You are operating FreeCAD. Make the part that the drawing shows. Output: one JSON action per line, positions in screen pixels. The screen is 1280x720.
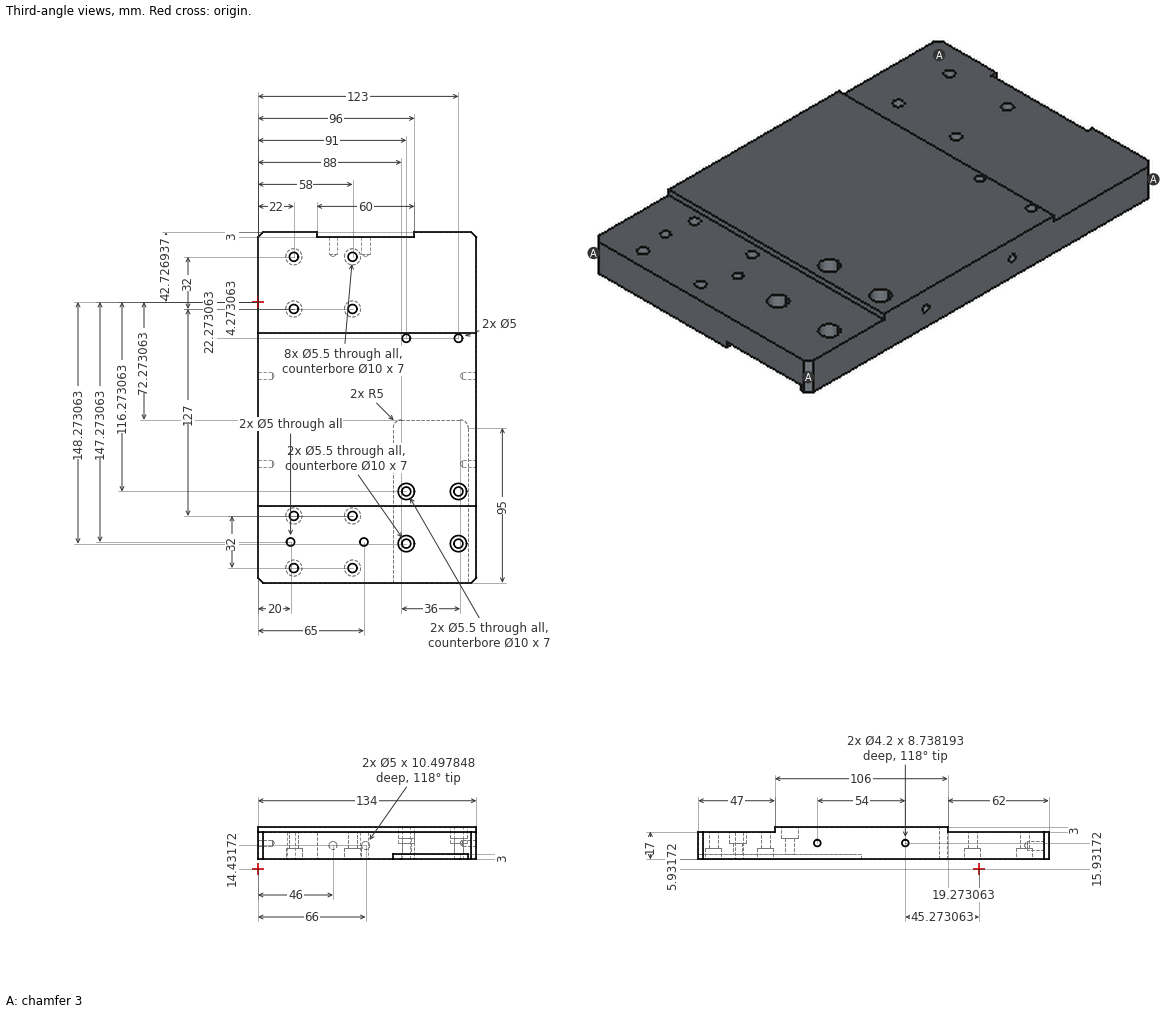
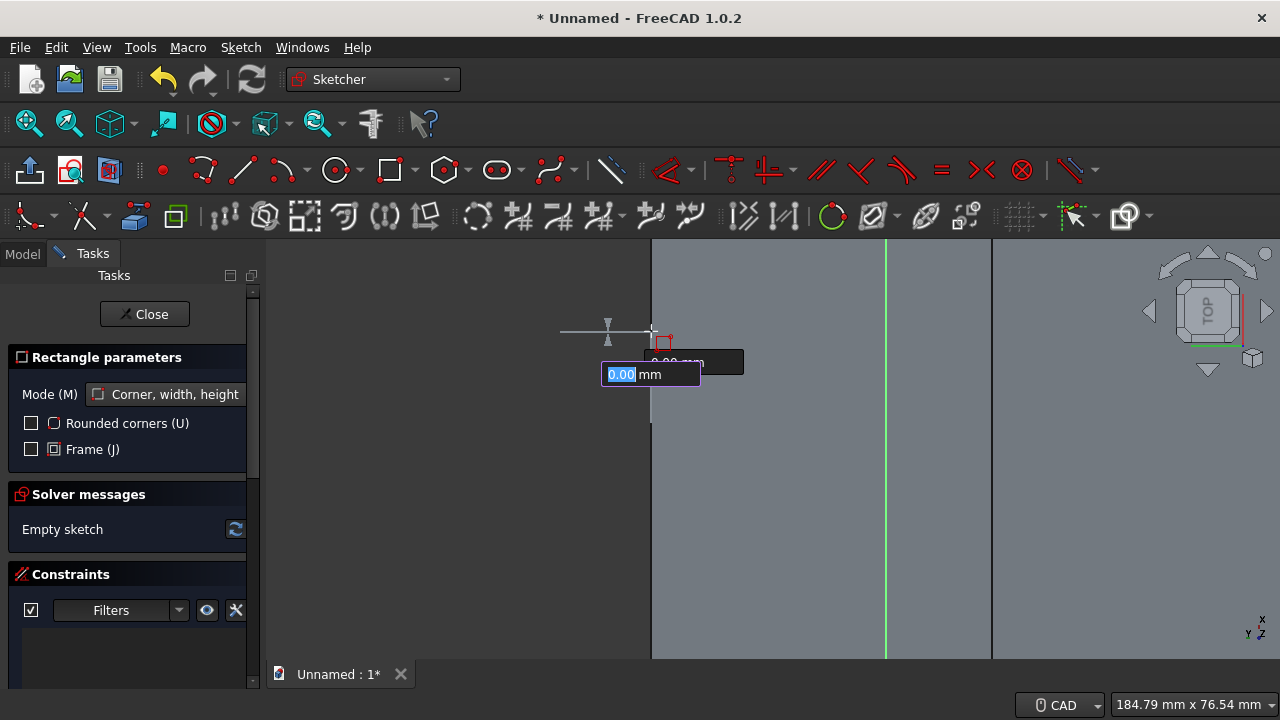
{"action": "scroll", "coordinate": [652, 331], "scroll_direction": "down", "scroll_amount": 4}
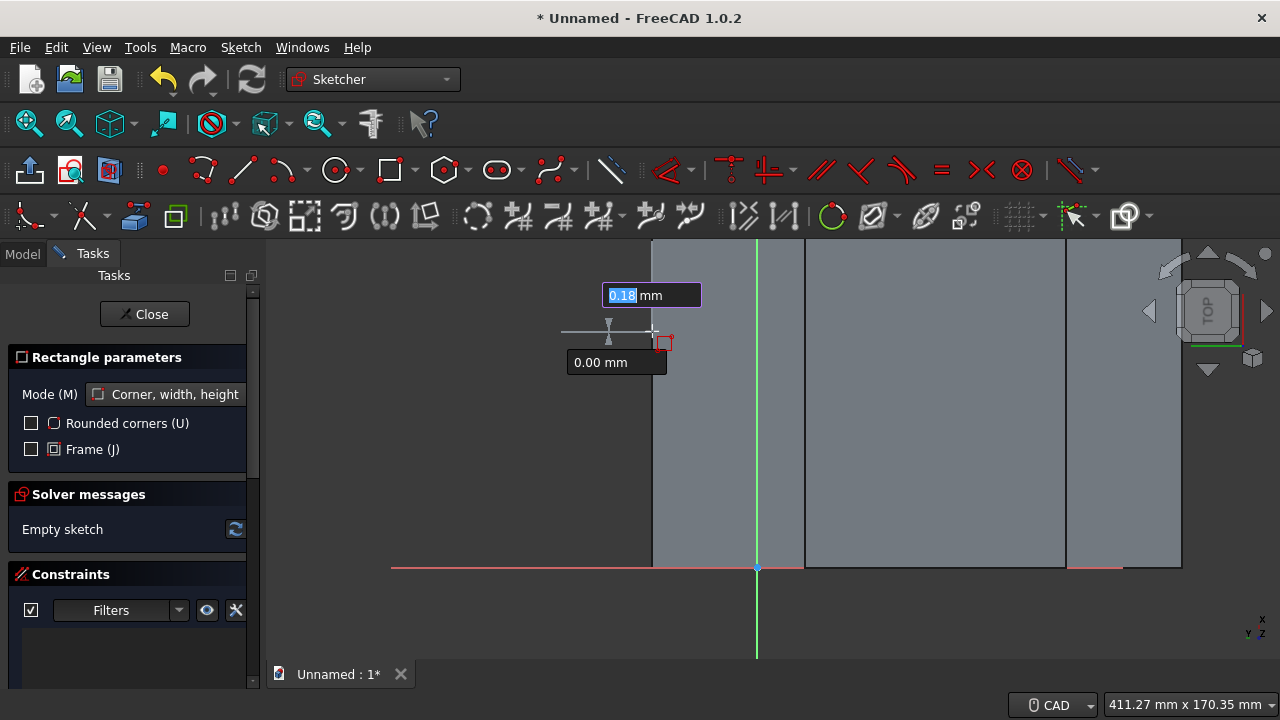
{"action": "left_click", "coordinate": [659, 479]}
{"action": "key", "text": "Escape"}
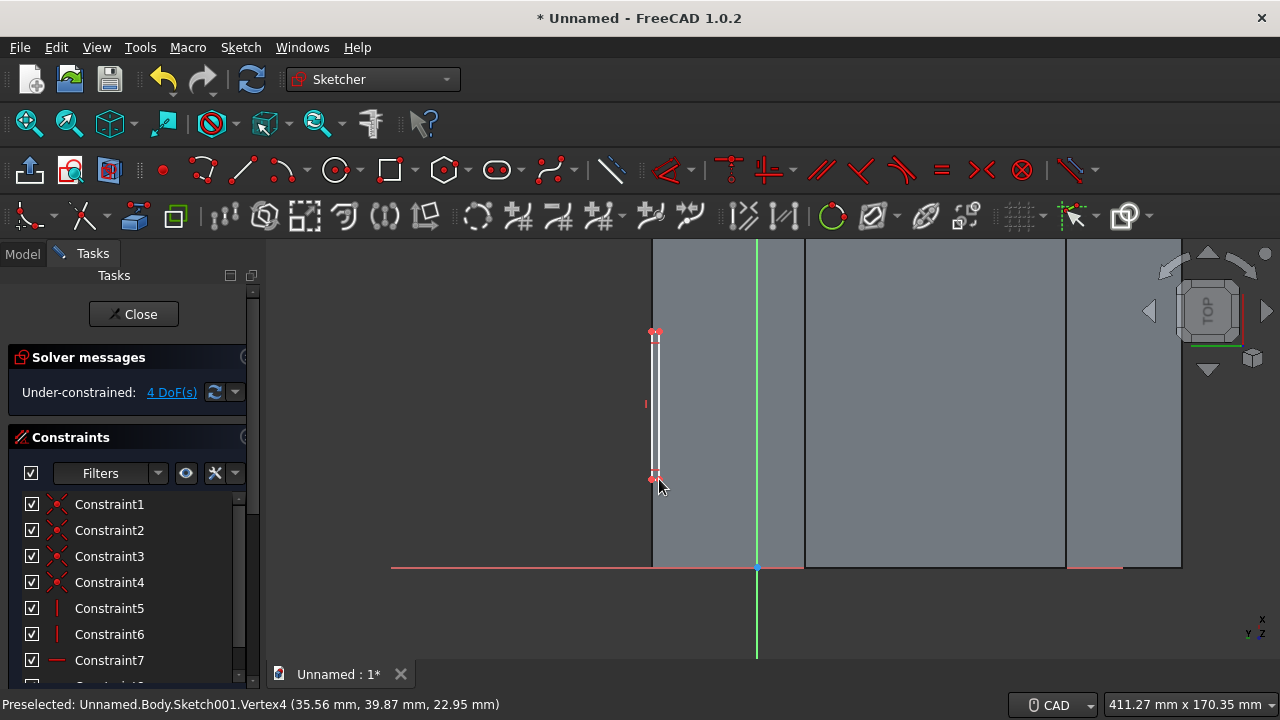
{"action": "left_click", "coordinate": [666, 170]}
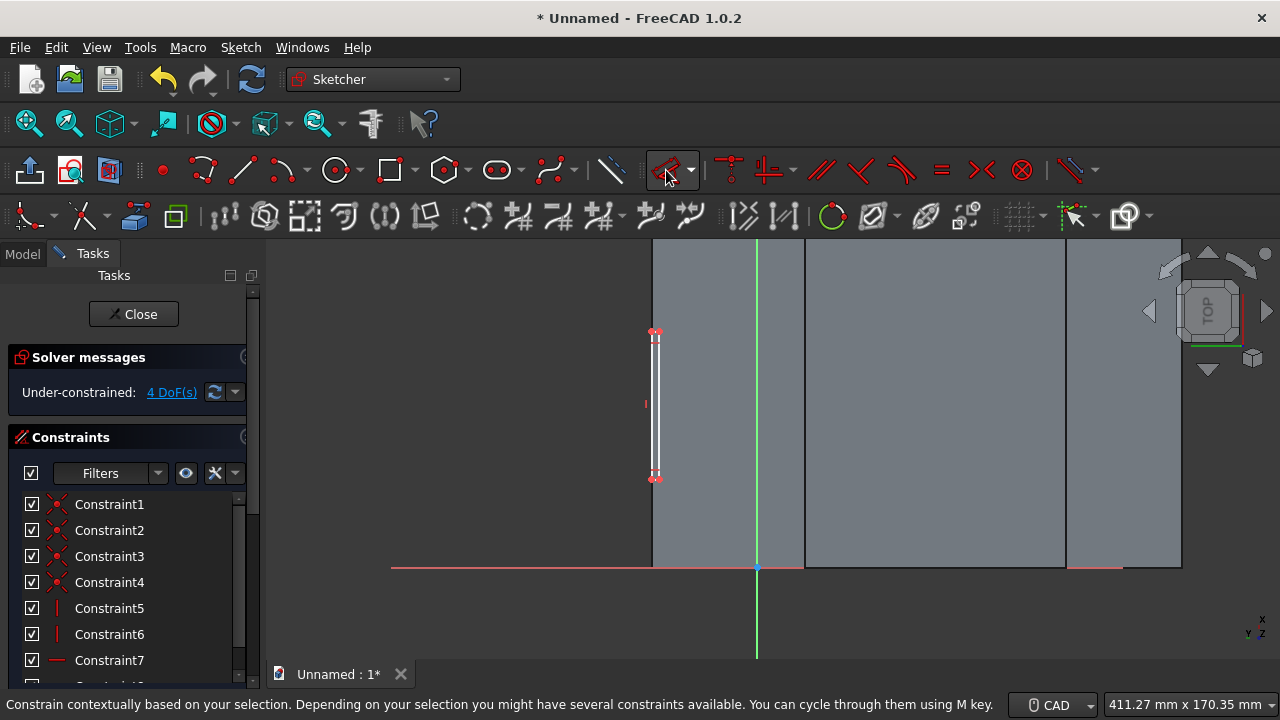
{"action": "scroll", "coordinate": [655, 480], "scroll_direction": "up", "scroll_amount": 9}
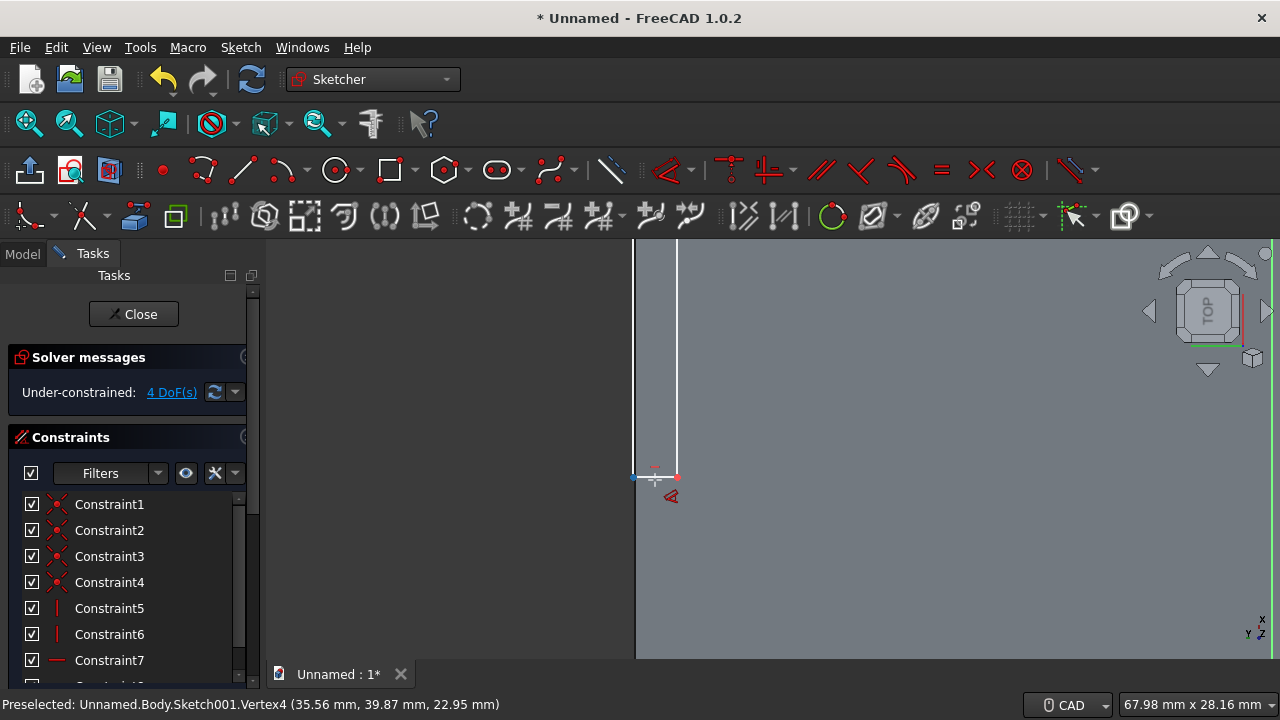
{"action": "left_click", "coordinate": [655, 477]}
{"action": "left_click", "coordinate": [655, 511]}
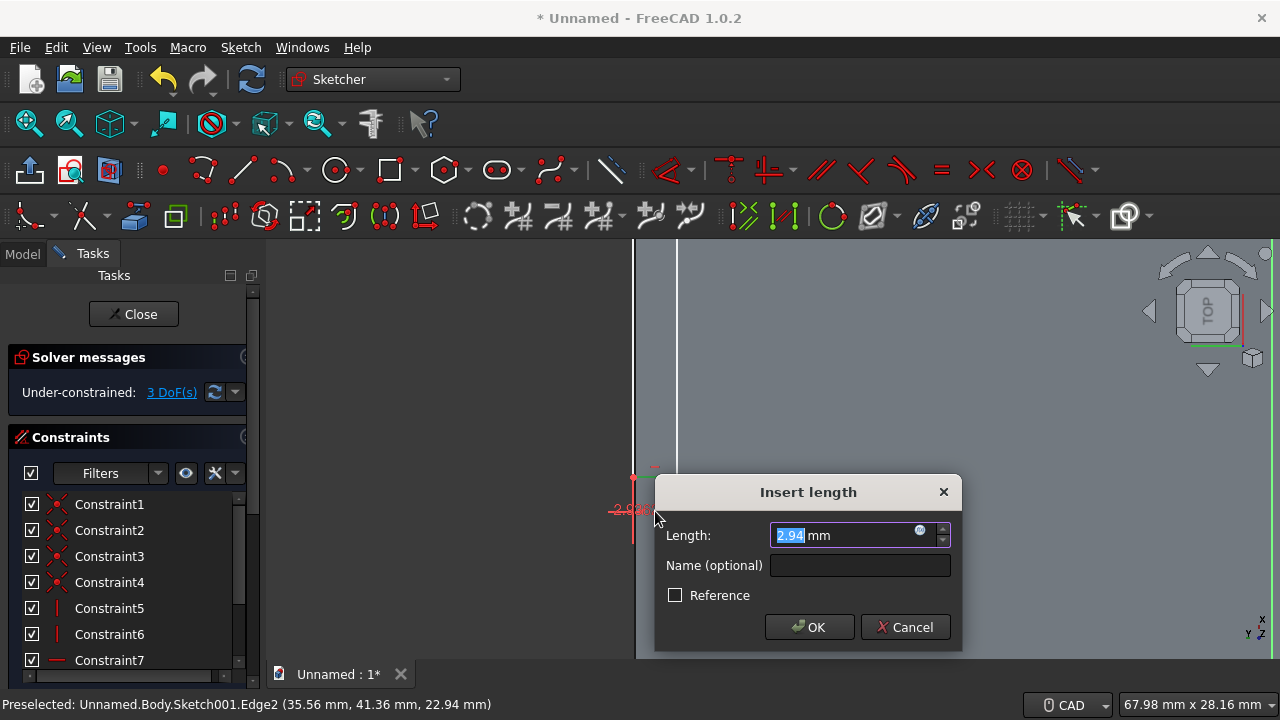
{"action": "type", "text": "3"}
{"action": "key", "text": "Return"}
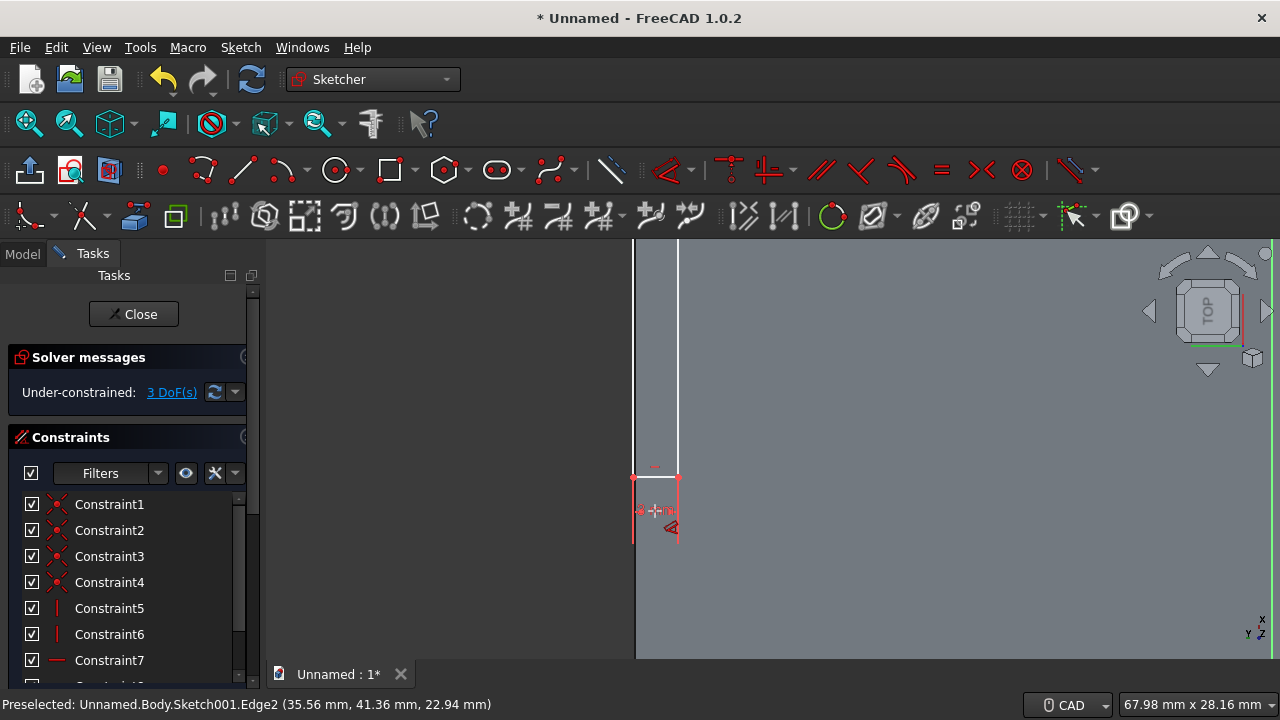
{"action": "scroll", "coordinate": [655, 480], "scroll_direction": "down", "scroll_amount": 9}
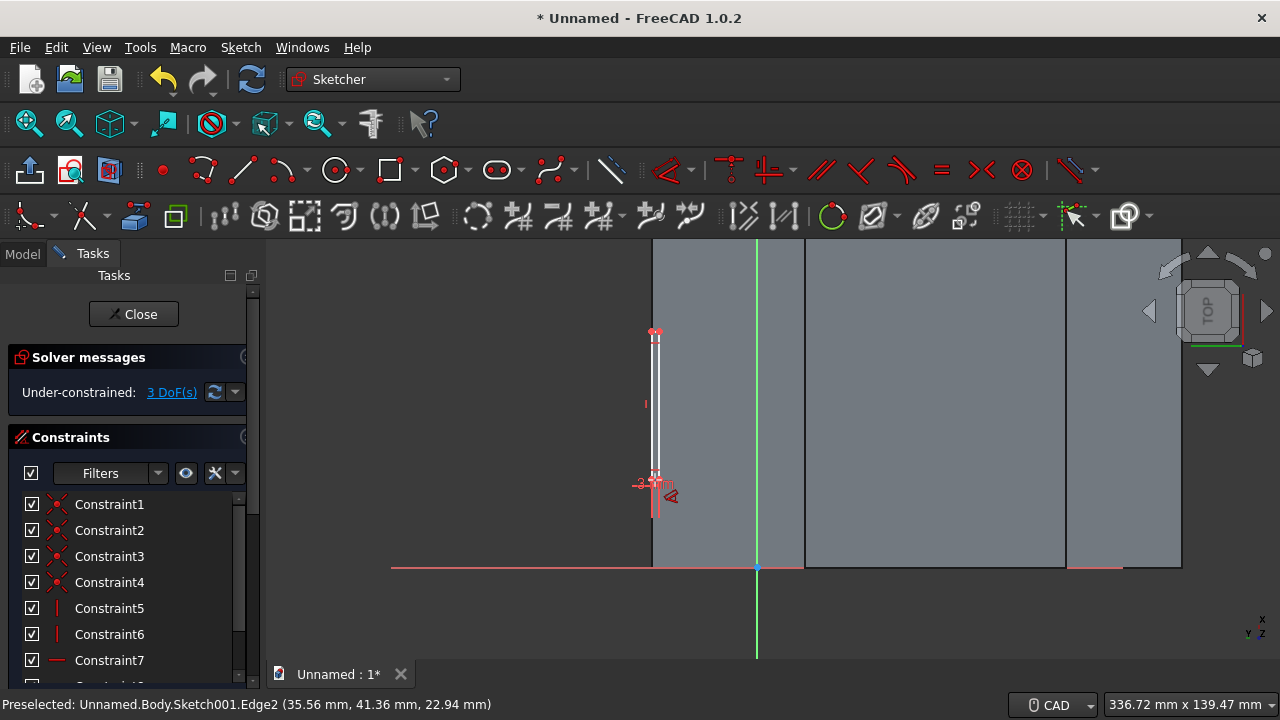
{"action": "scroll", "coordinate": [652, 450], "scroll_direction": "up", "scroll_amount": 4}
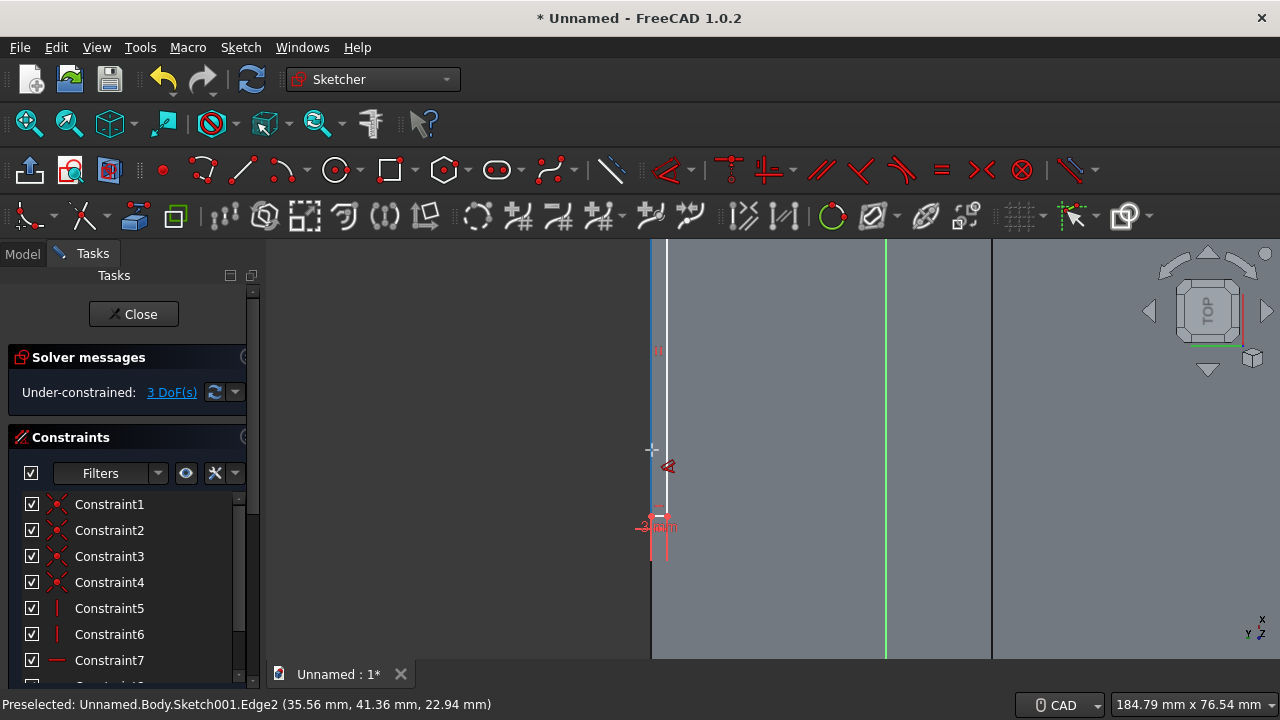
{"action": "left_click", "coordinate": [651, 450]}
{"action": "left_click", "coordinate": [617, 392]}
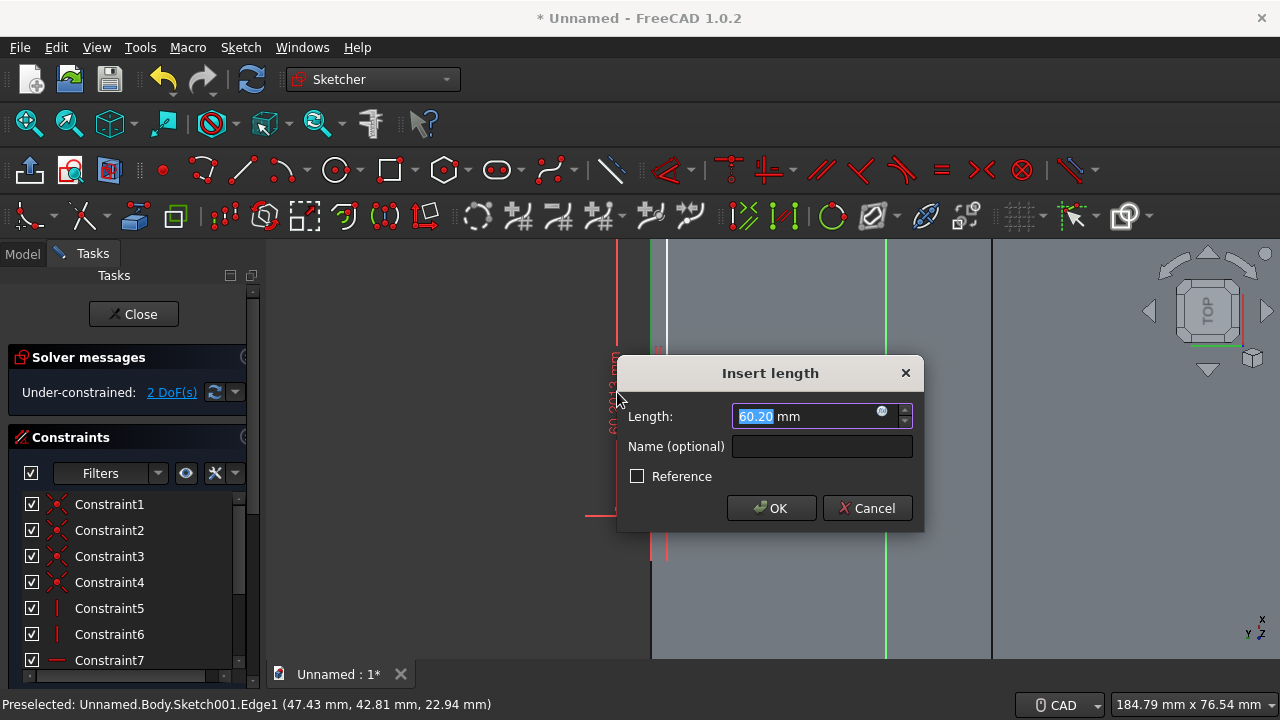
{"action": "type", "text": "60"}
{"action": "key", "text": "Return"}